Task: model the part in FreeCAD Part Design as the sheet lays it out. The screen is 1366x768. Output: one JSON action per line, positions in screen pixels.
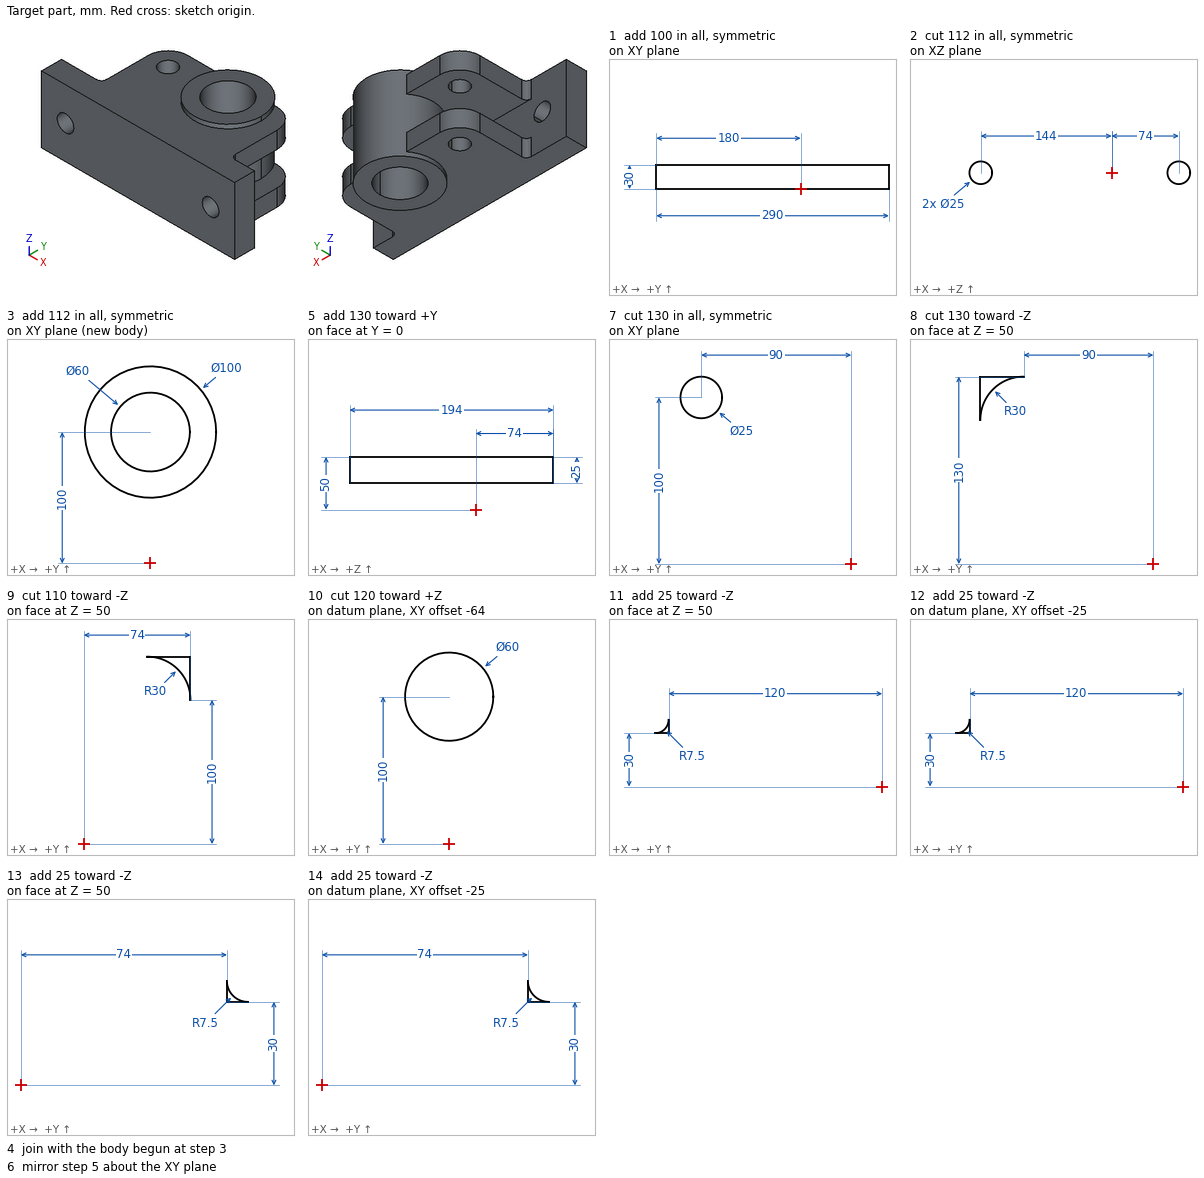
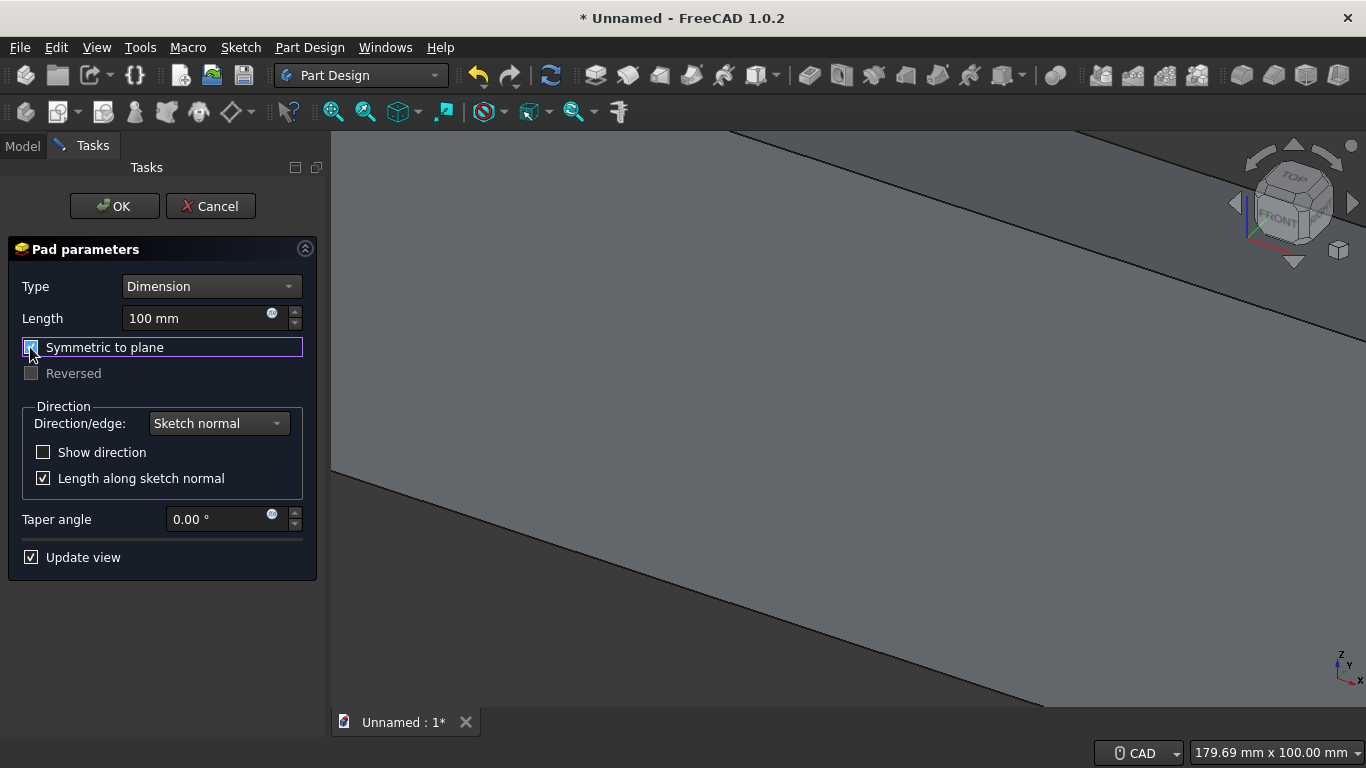
{"action": "left_click", "coordinate": [115, 206]}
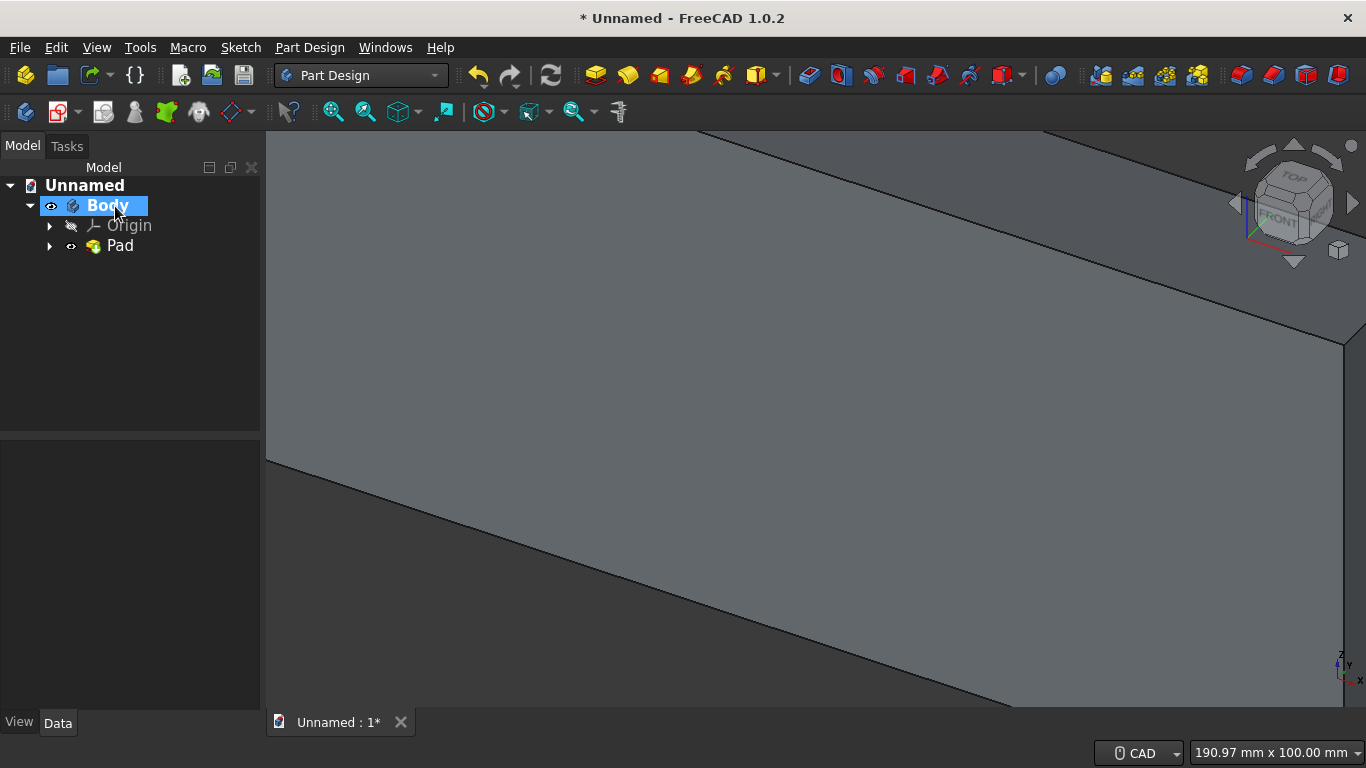
{"action": "left_click", "coordinate": [334, 112]}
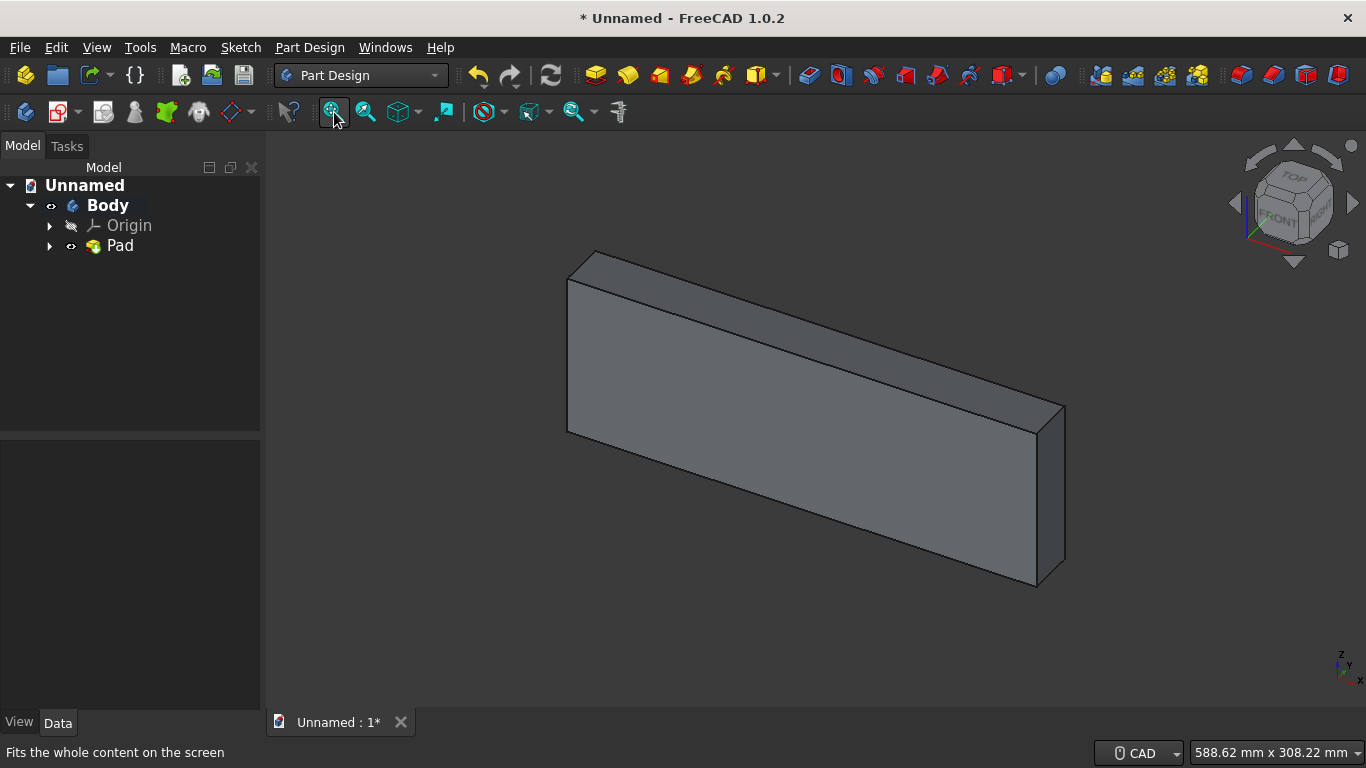
{"action": "left_click", "coordinate": [58, 112]}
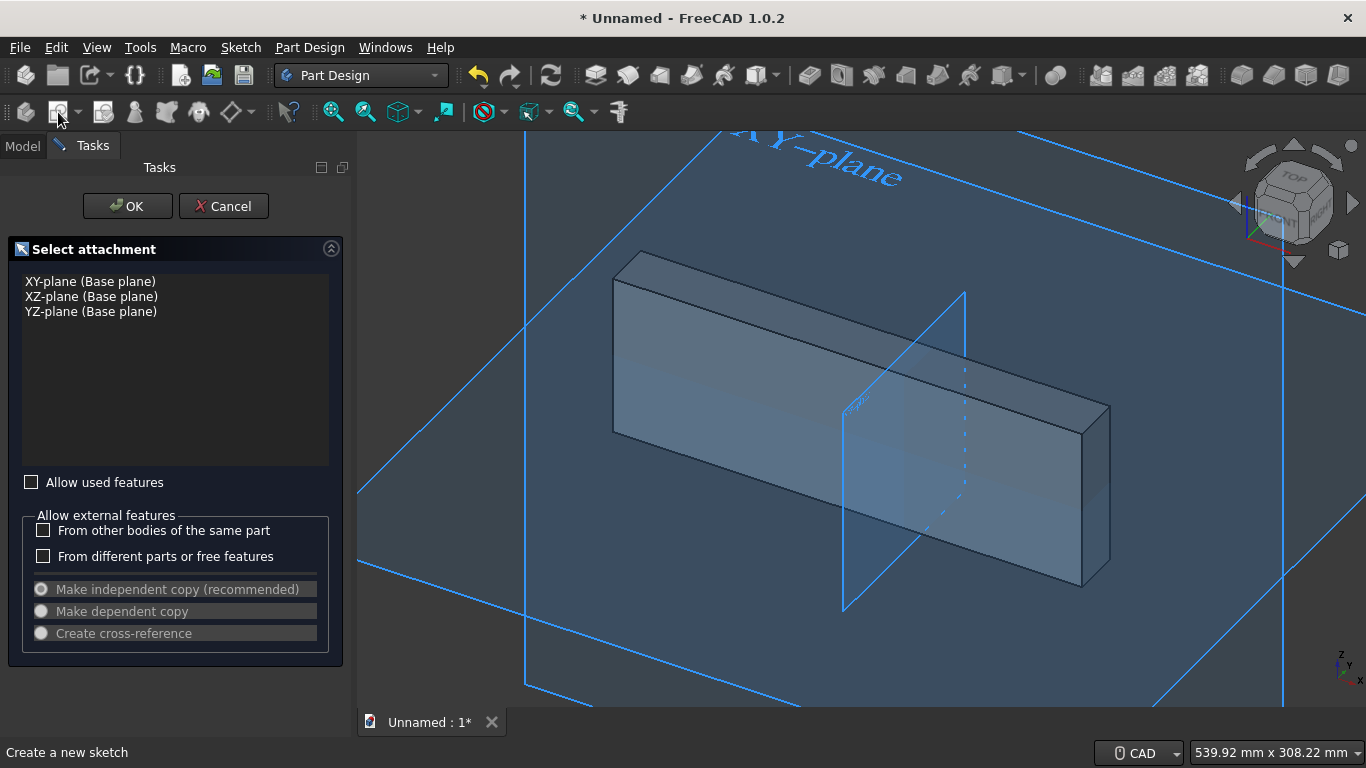
{"action": "left_click", "coordinate": [82, 296]}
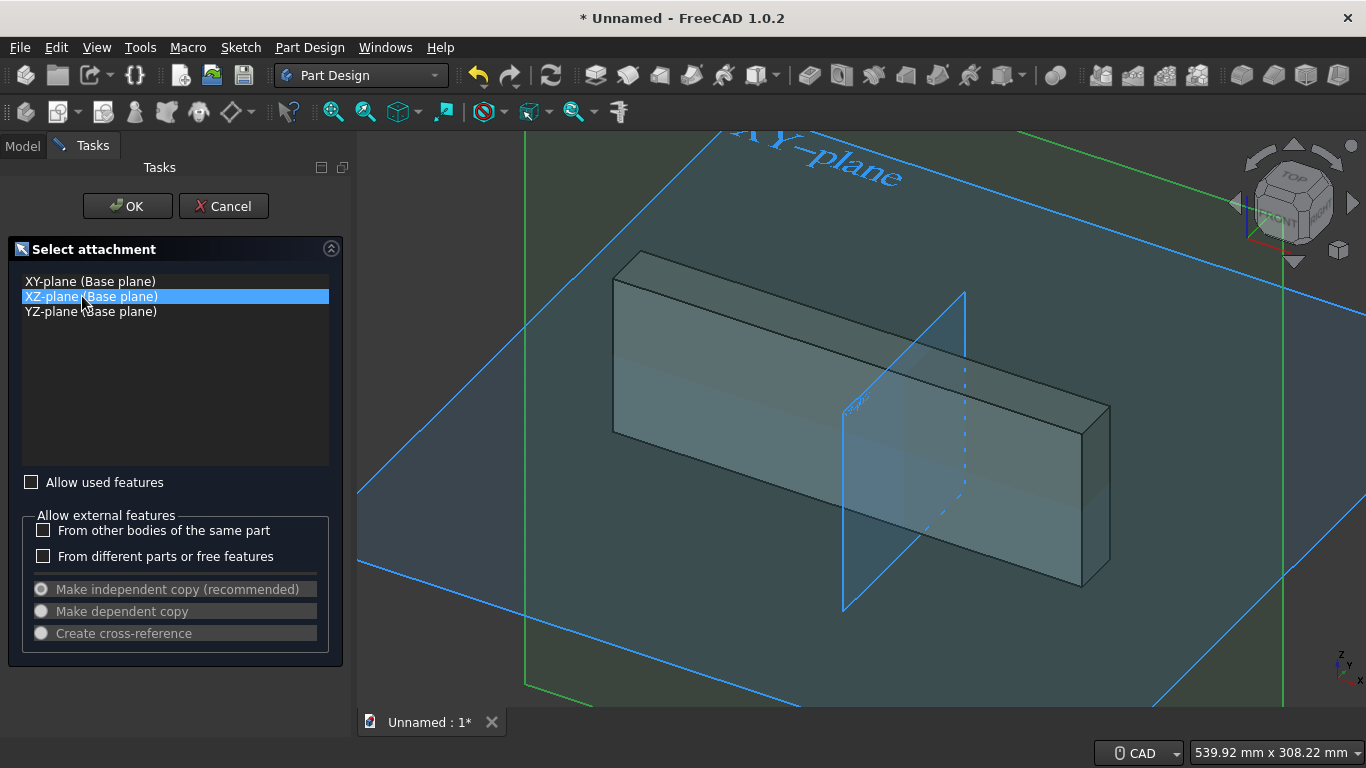
{"action": "left_click", "coordinate": [128, 206]}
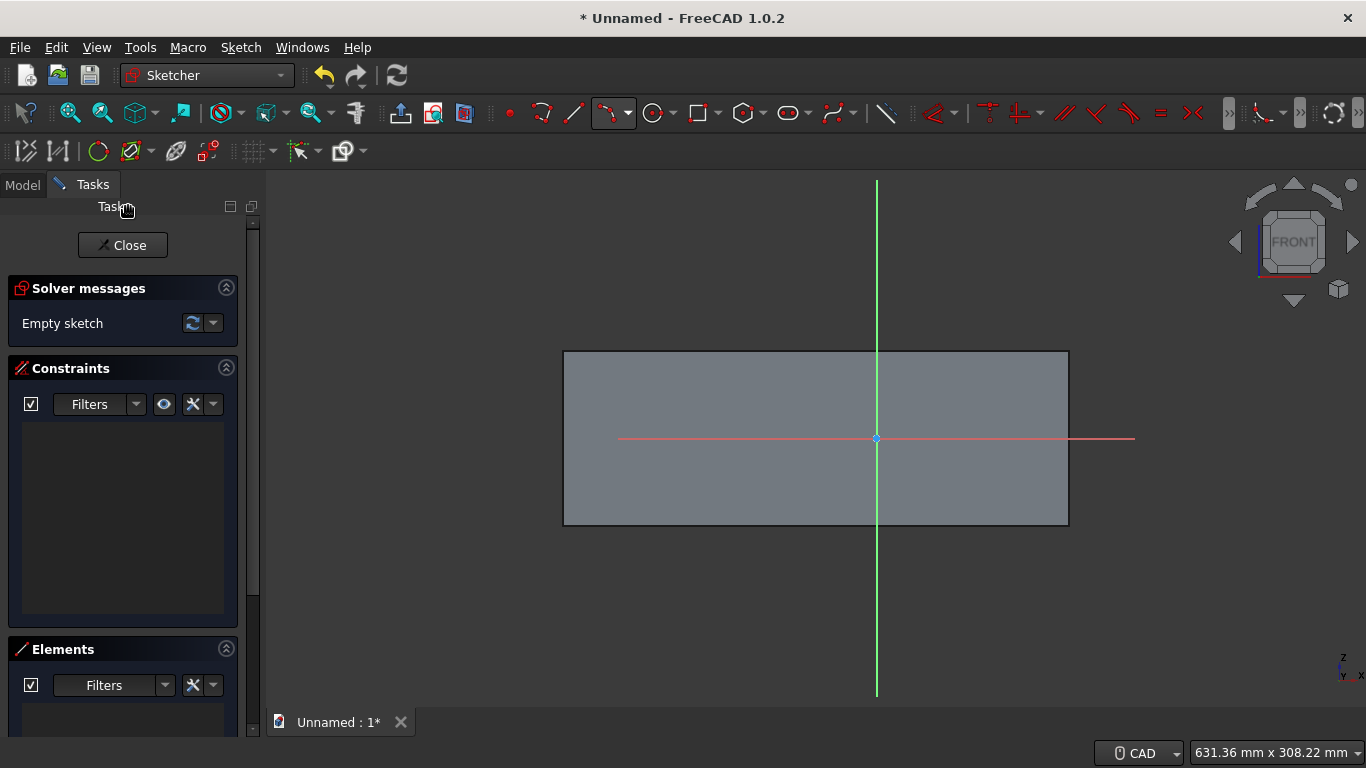
{"action": "scroll", "coordinate": [955, 439], "scroll_direction": "up", "scroll_amount": 2}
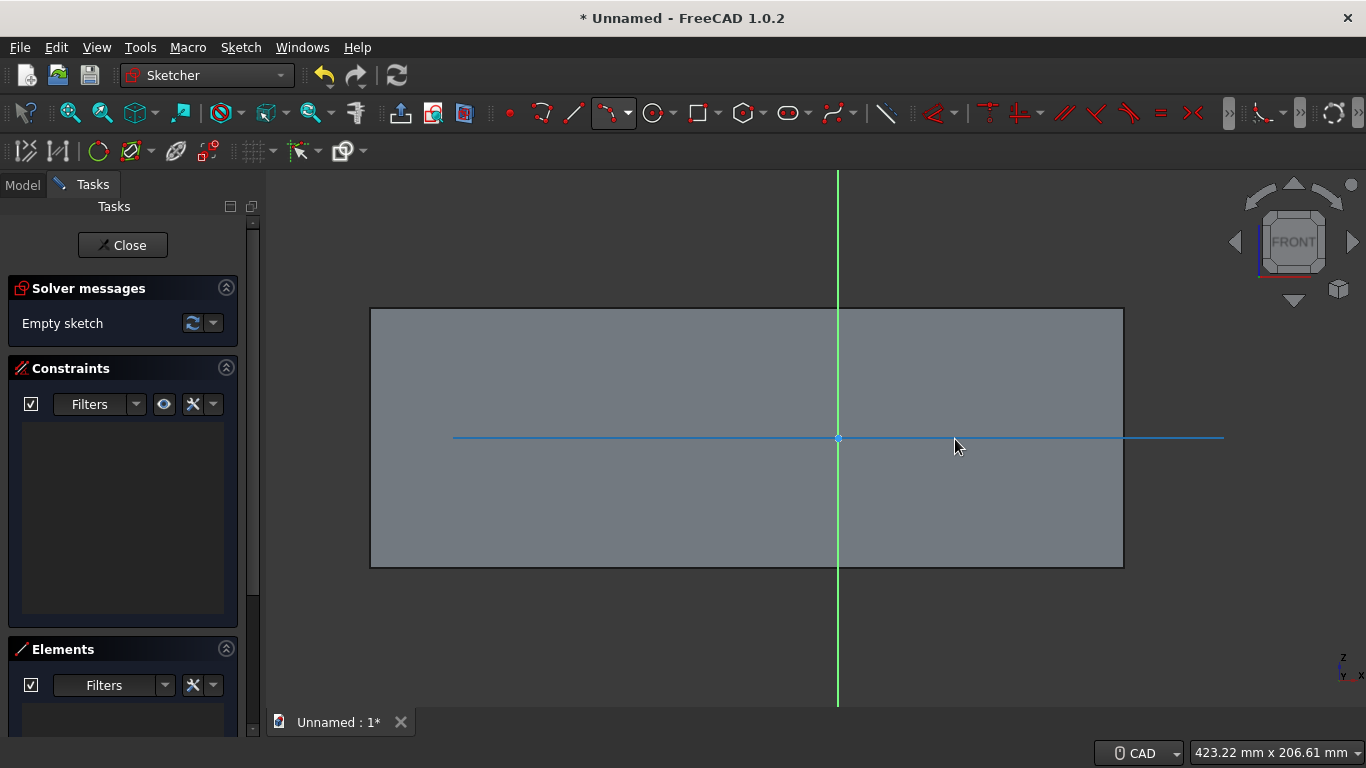
{"action": "left_click", "coordinate": [654, 114]}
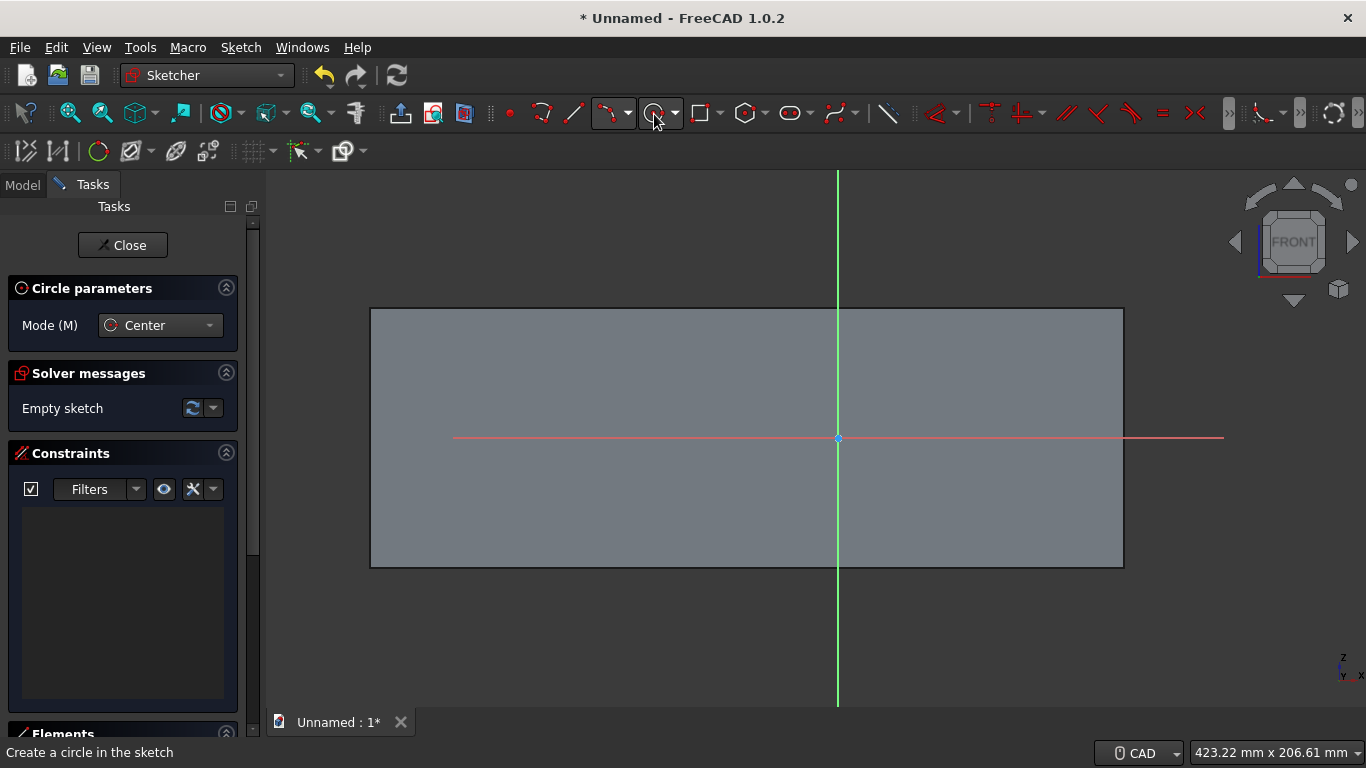
{"action": "left_click", "coordinate": [464, 438]}
{"action": "mouse_move", "coordinate": [487, 415]}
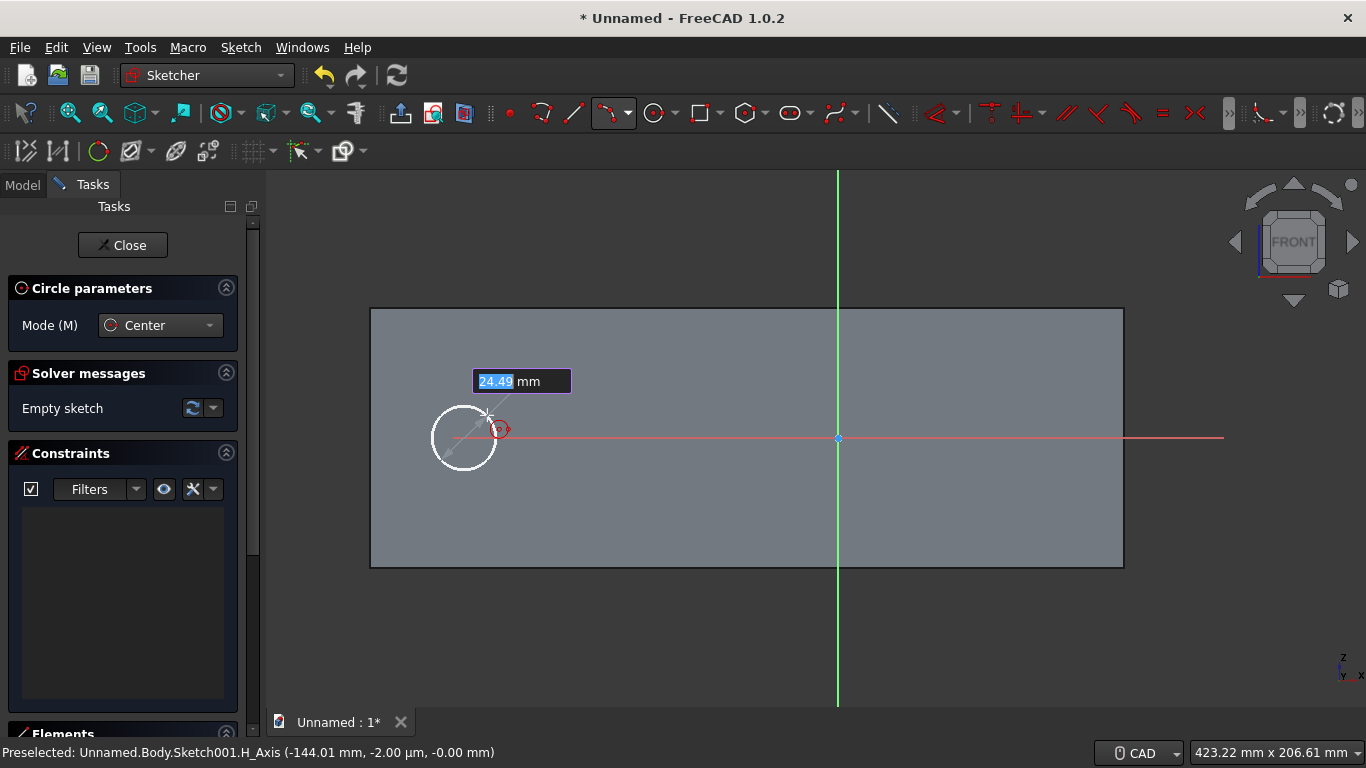
{"action": "type", "text": "25"}
{"action": "key", "text": "Return"}